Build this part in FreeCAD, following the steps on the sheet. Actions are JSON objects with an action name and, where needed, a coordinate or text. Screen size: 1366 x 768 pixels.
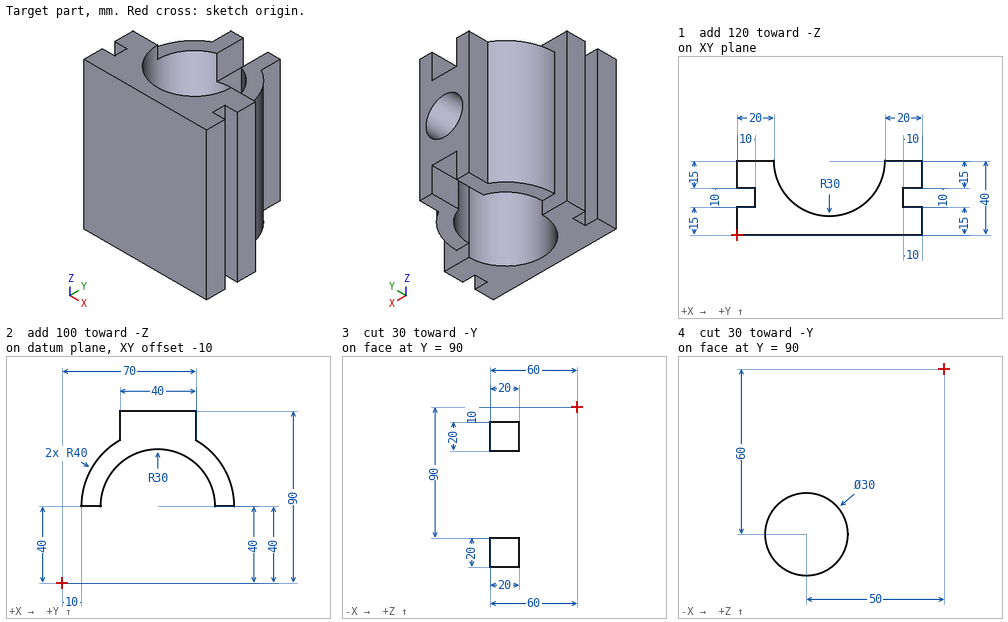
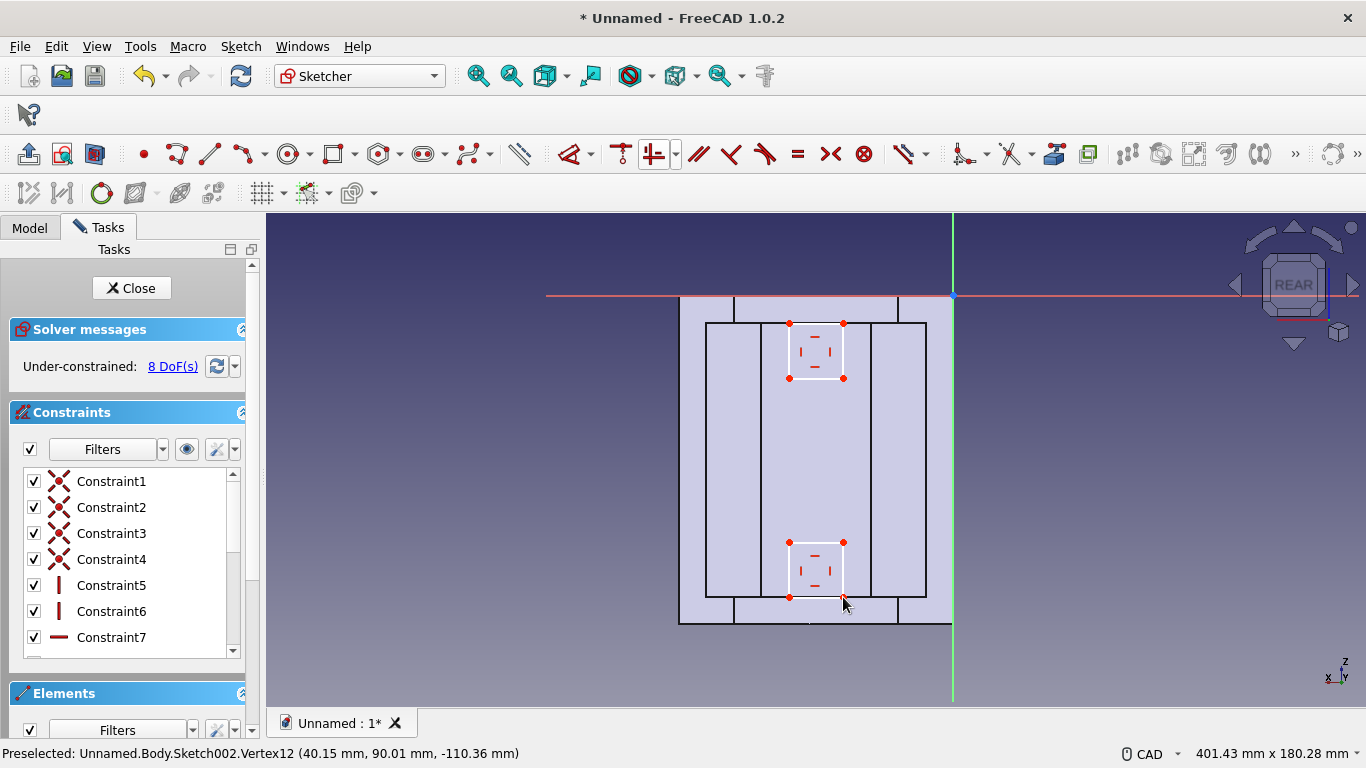
{"action": "left_click", "coordinate": [568, 154]}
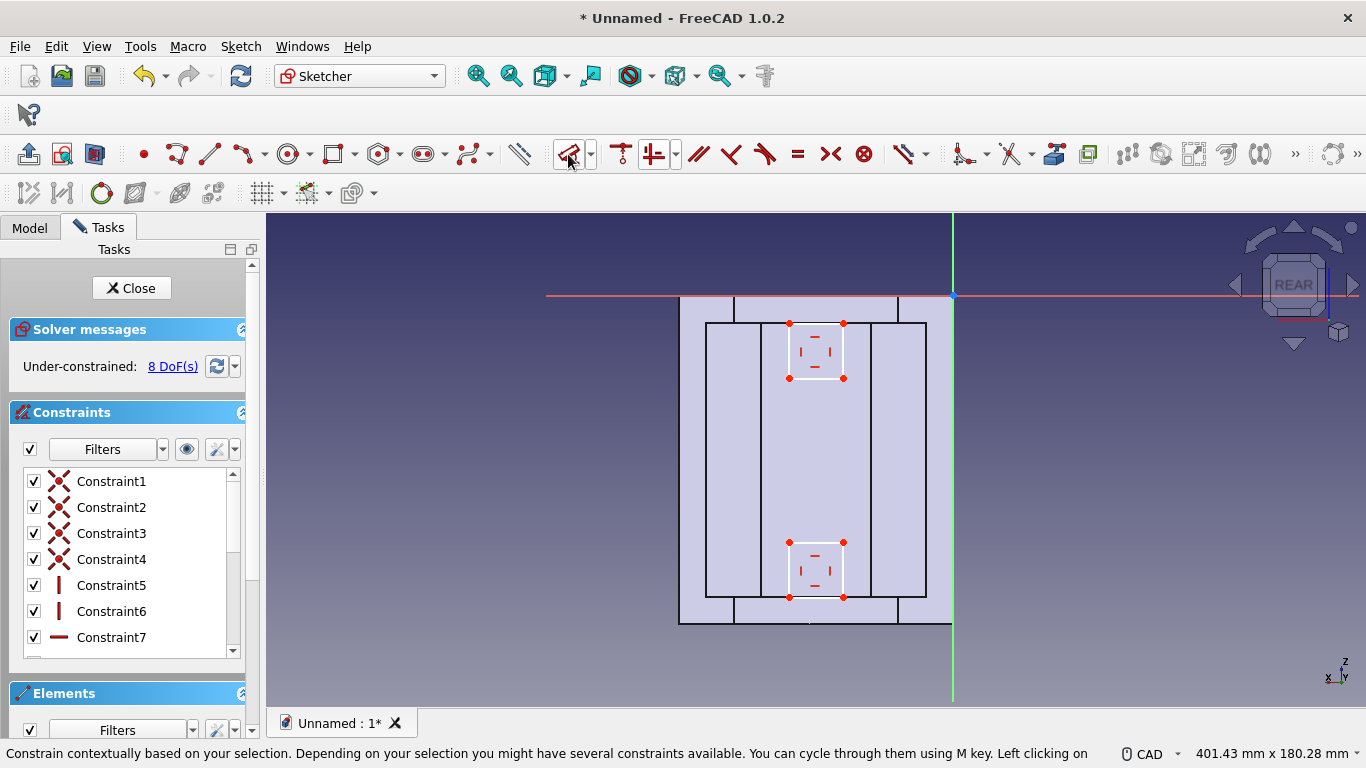
{"action": "left_click", "coordinate": [789, 340]}
{"action": "left_click", "coordinate": [755, 351]}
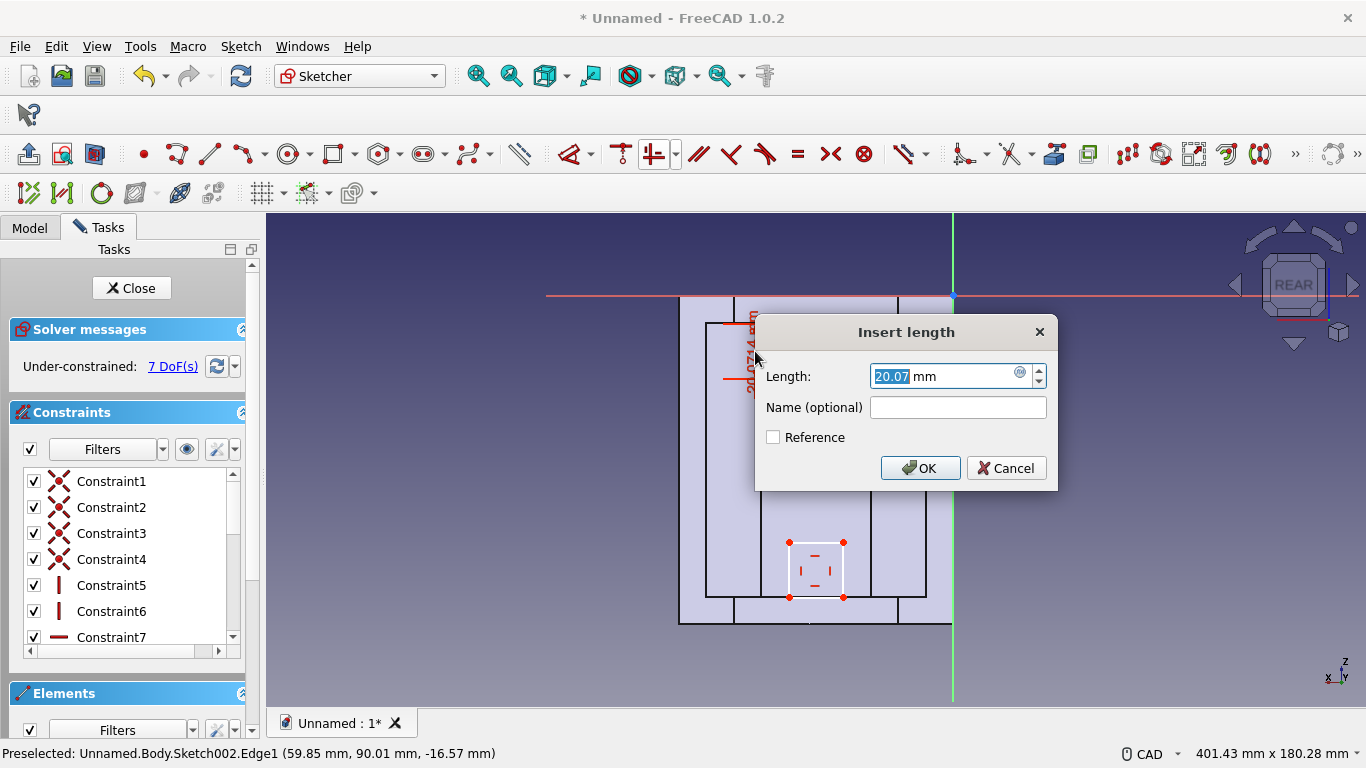
{"action": "type", "text": "20"}
{"action": "key", "text": "Return"}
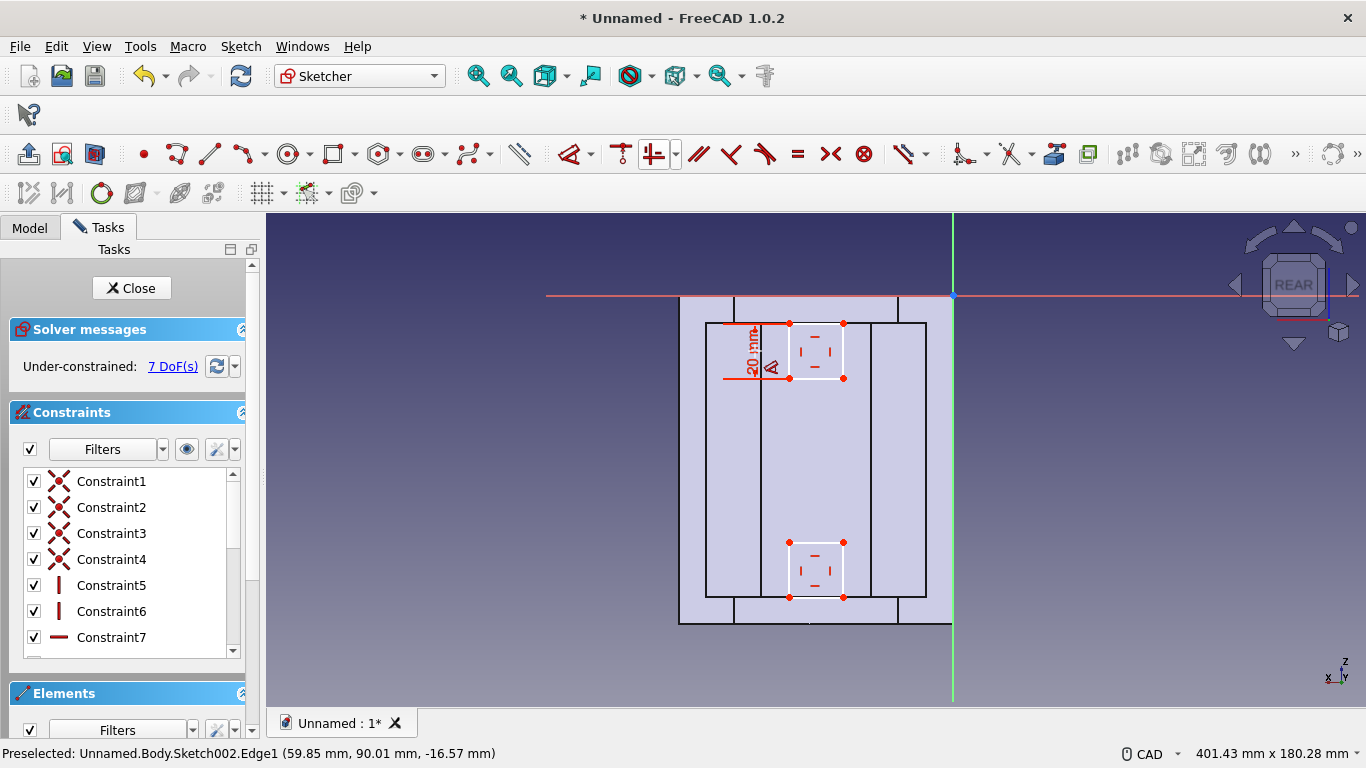
{"action": "left_click", "coordinate": [805, 379]}
{"action": "left_click", "coordinate": [828, 345]}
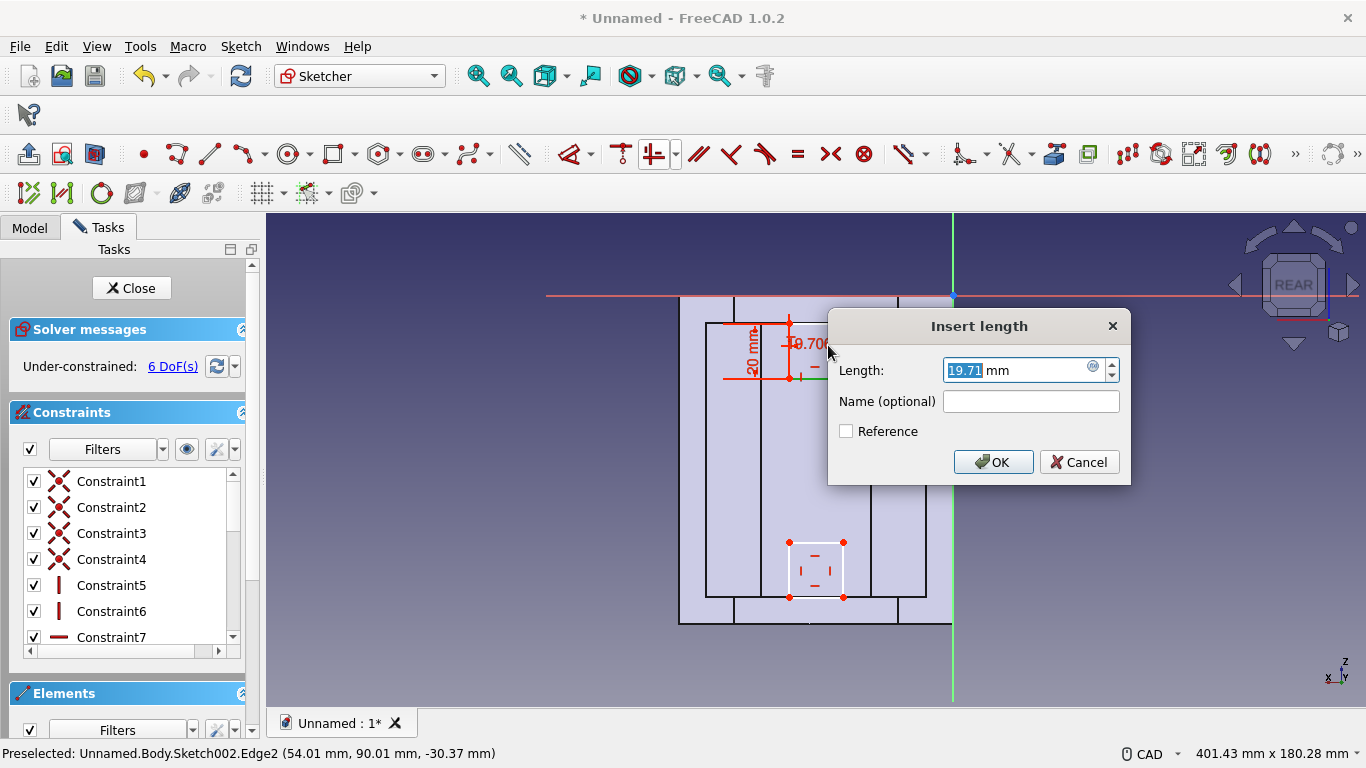
{"action": "type", "text": "20"}
{"action": "key", "text": "Return"}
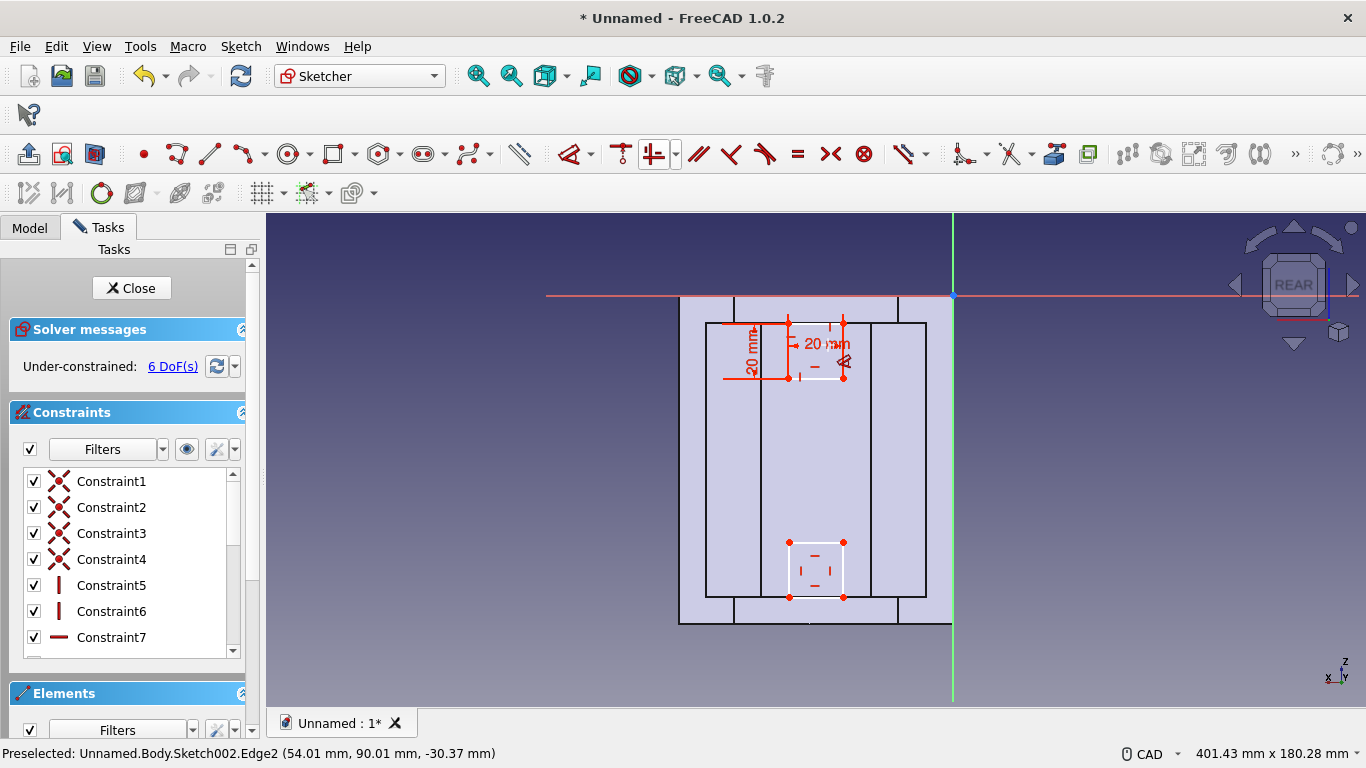
{"action": "left_click", "coordinate": [789, 559]}
{"action": "left_click", "coordinate": [755, 570]}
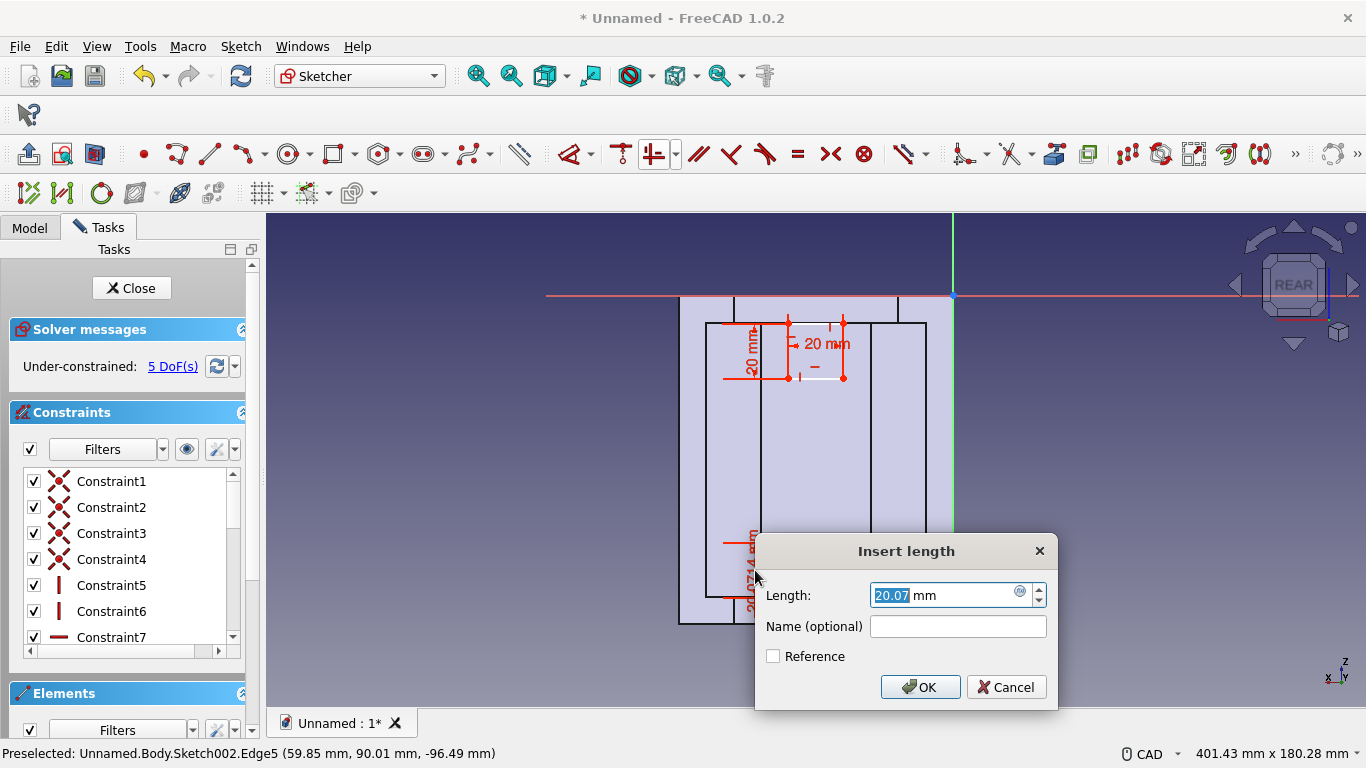
{"action": "type", "text": "20"}
{"action": "key", "text": "Return"}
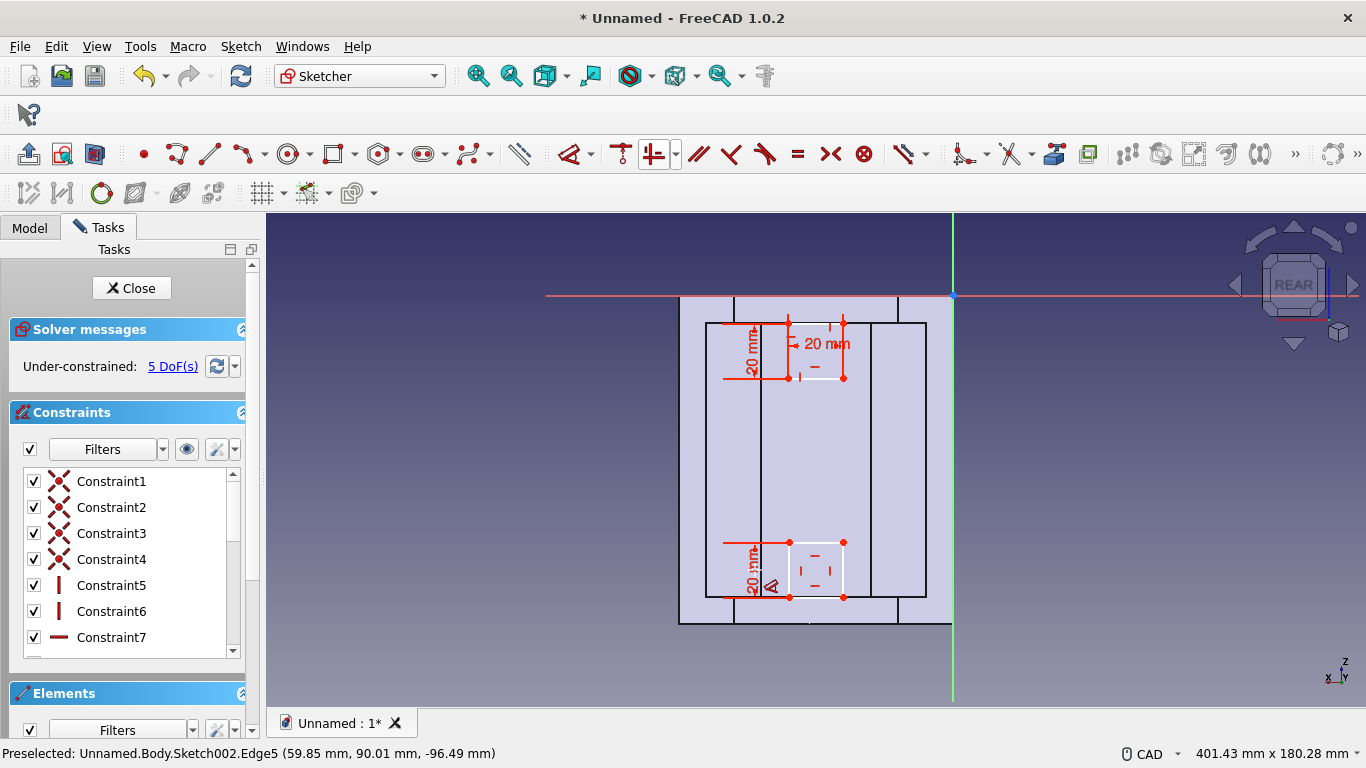
{"action": "left_click", "coordinate": [805, 598]}
{"action": "left_click", "coordinate": [816, 632]}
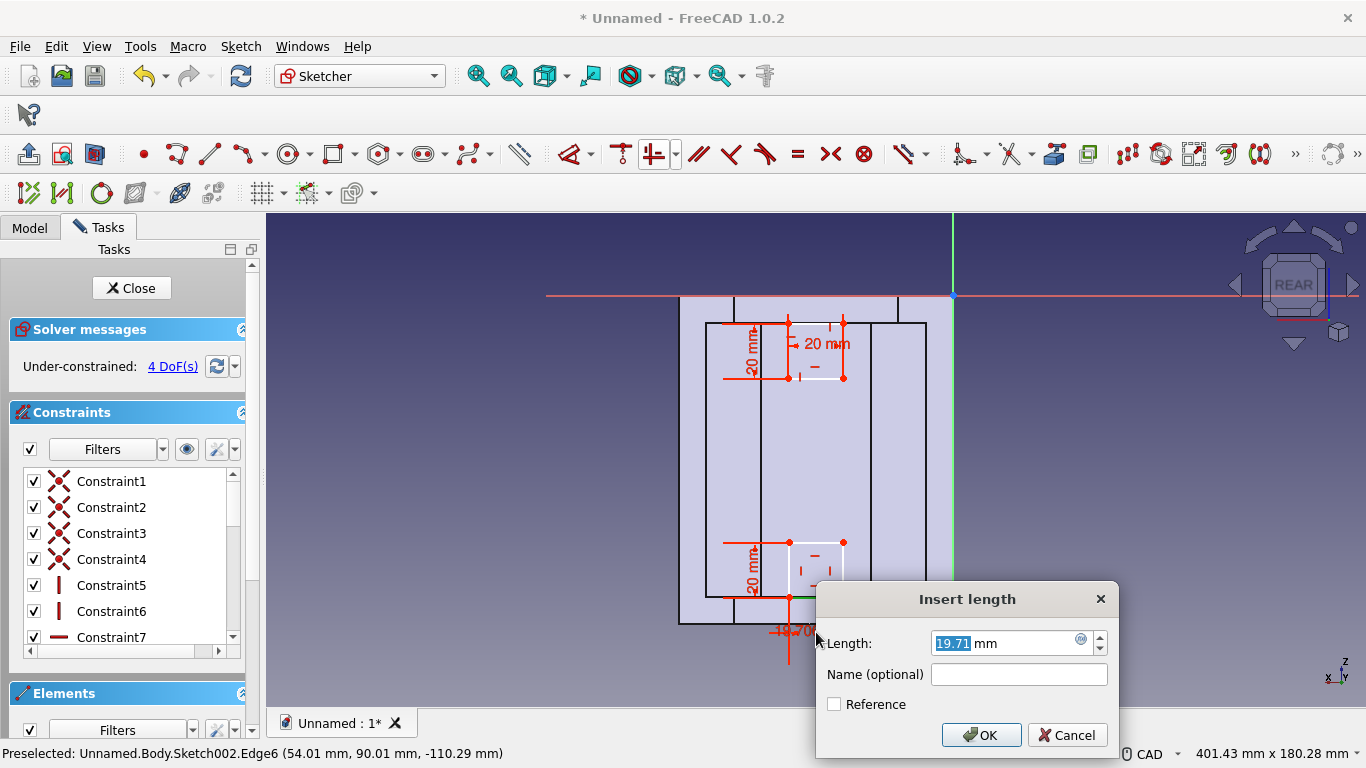
{"action": "type", "text": "20"}
{"action": "key", "text": "Return"}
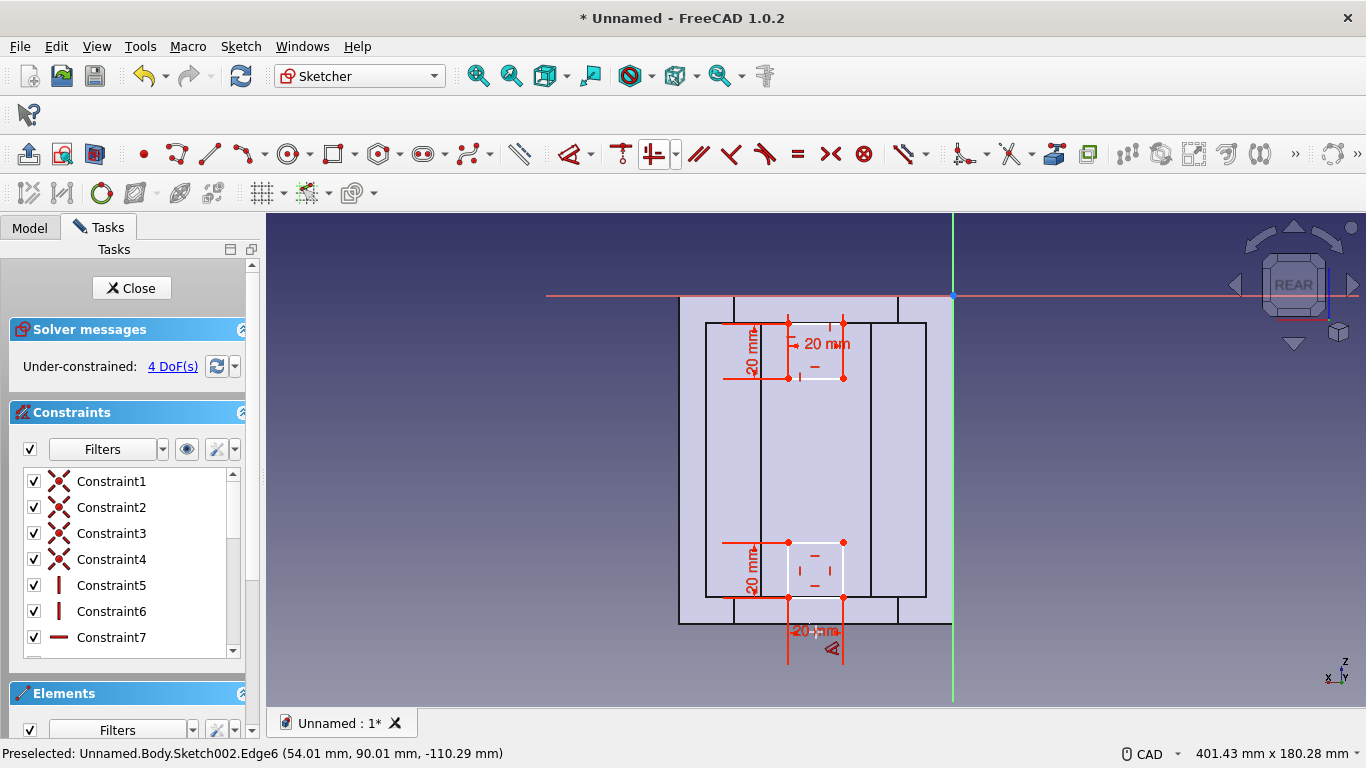
{"action": "left_click", "coordinate": [788, 324]}
{"action": "left_click", "coordinate": [871, 262]}